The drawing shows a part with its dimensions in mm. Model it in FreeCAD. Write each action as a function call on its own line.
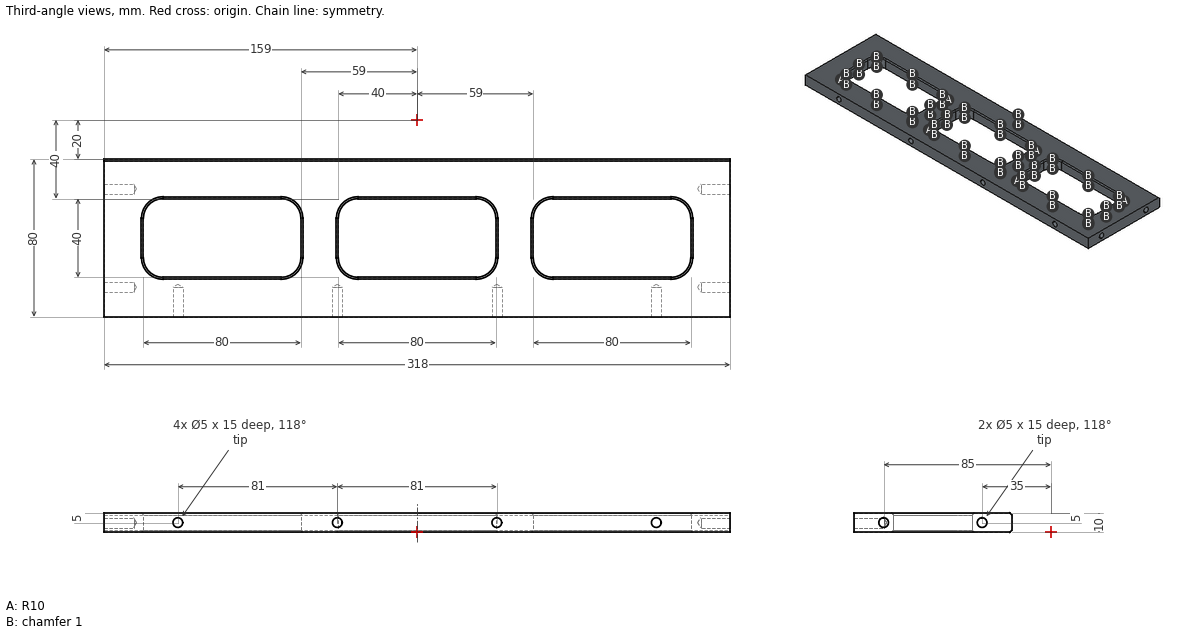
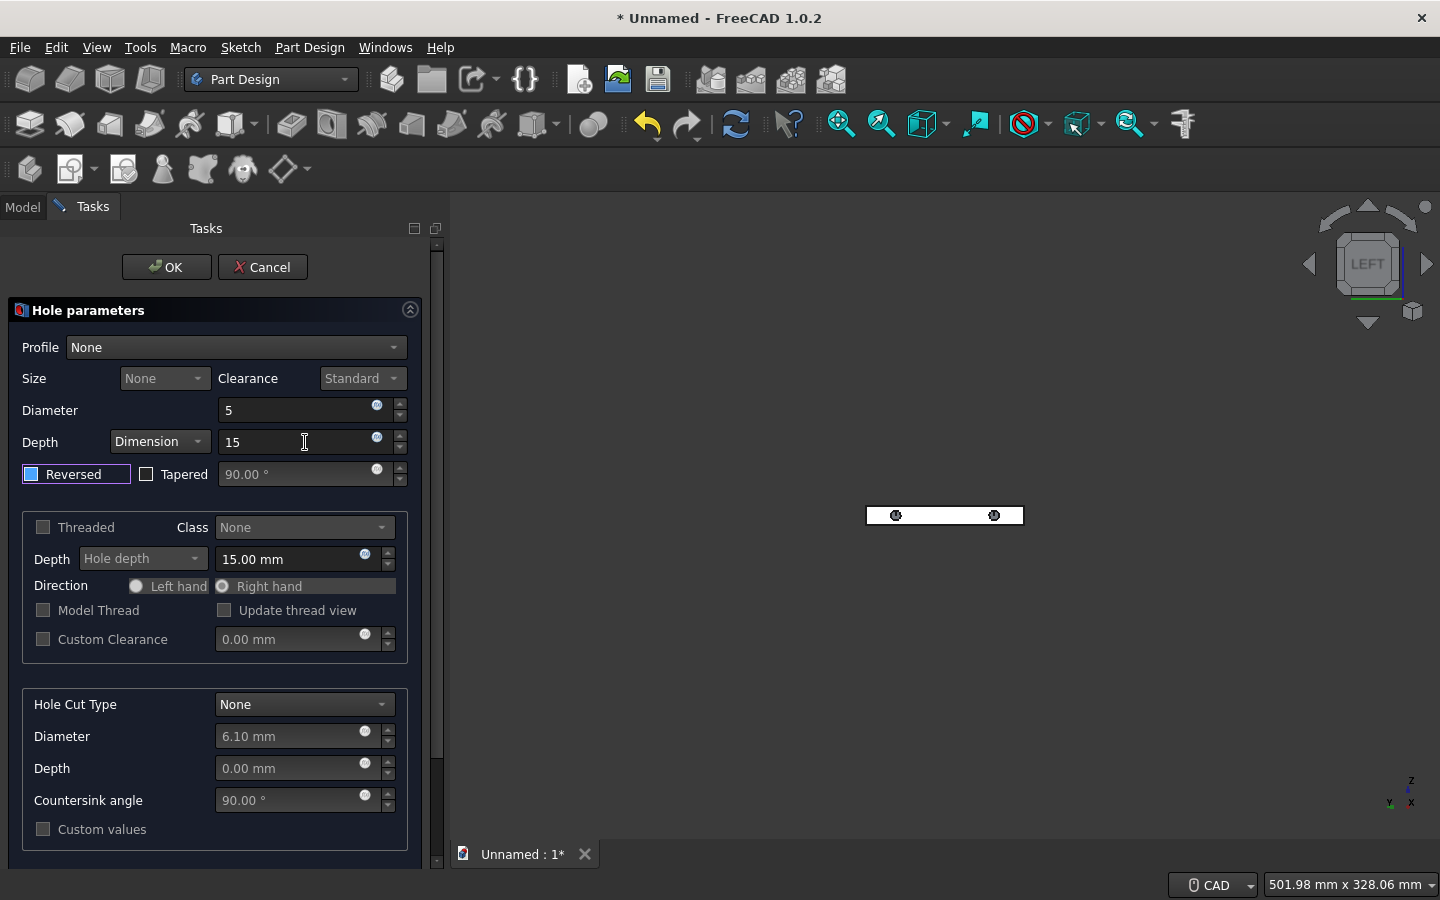
click(167, 267)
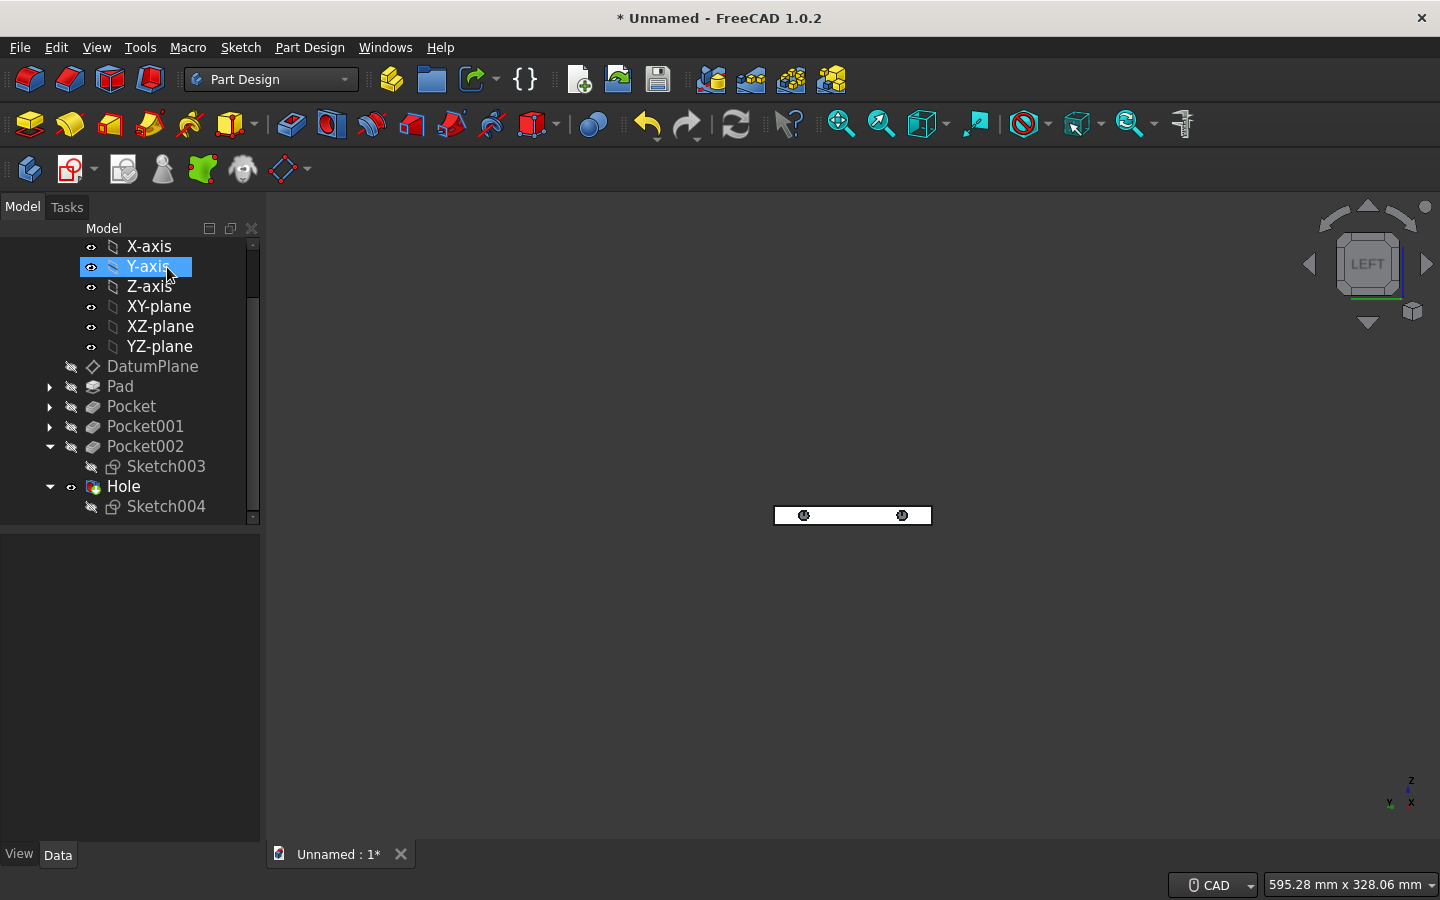
click(842, 124)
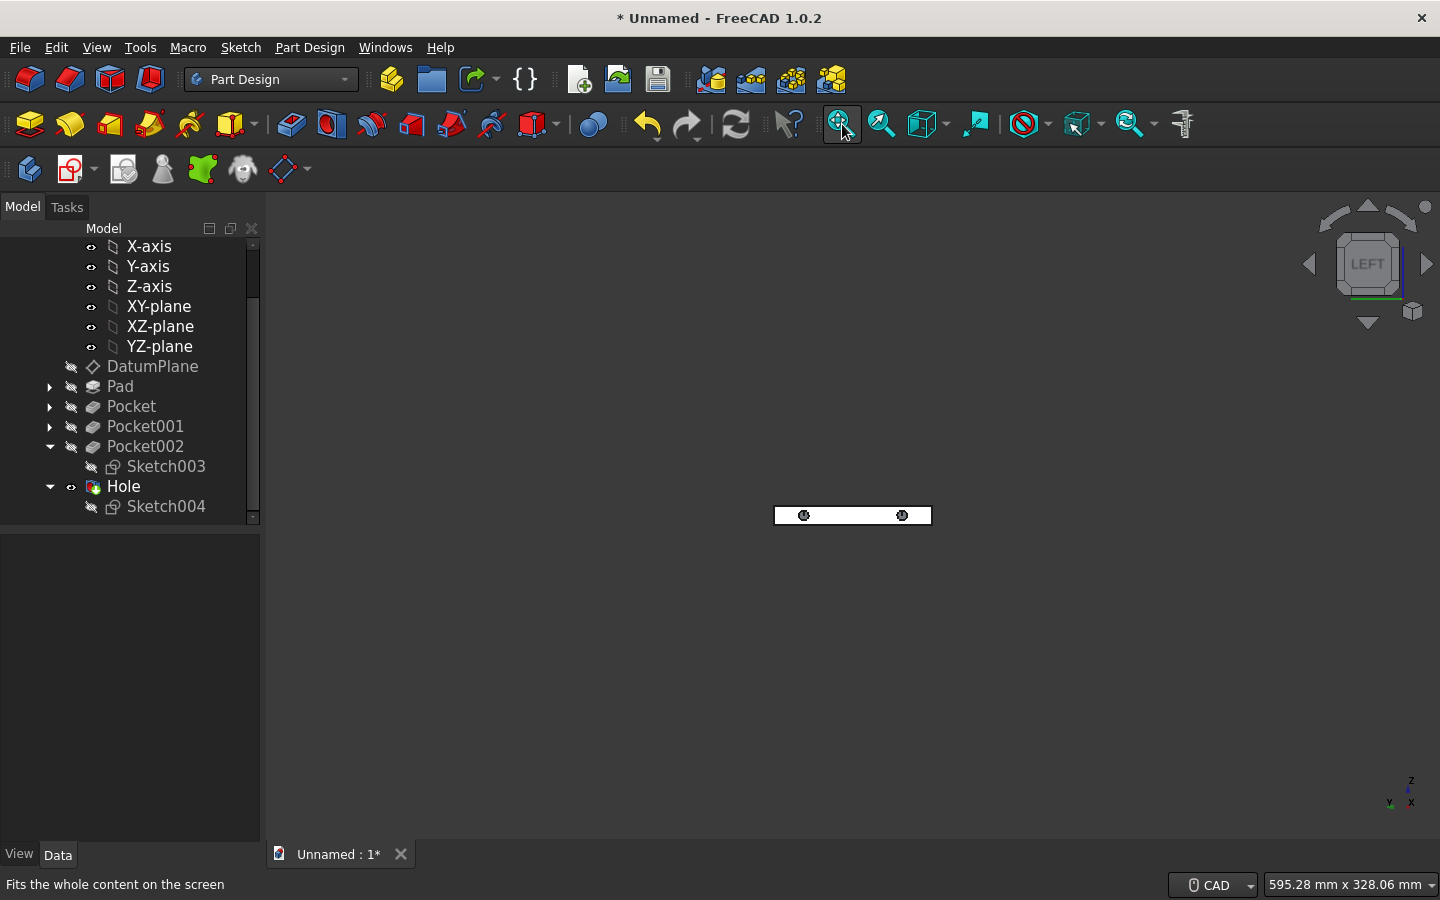
key(0)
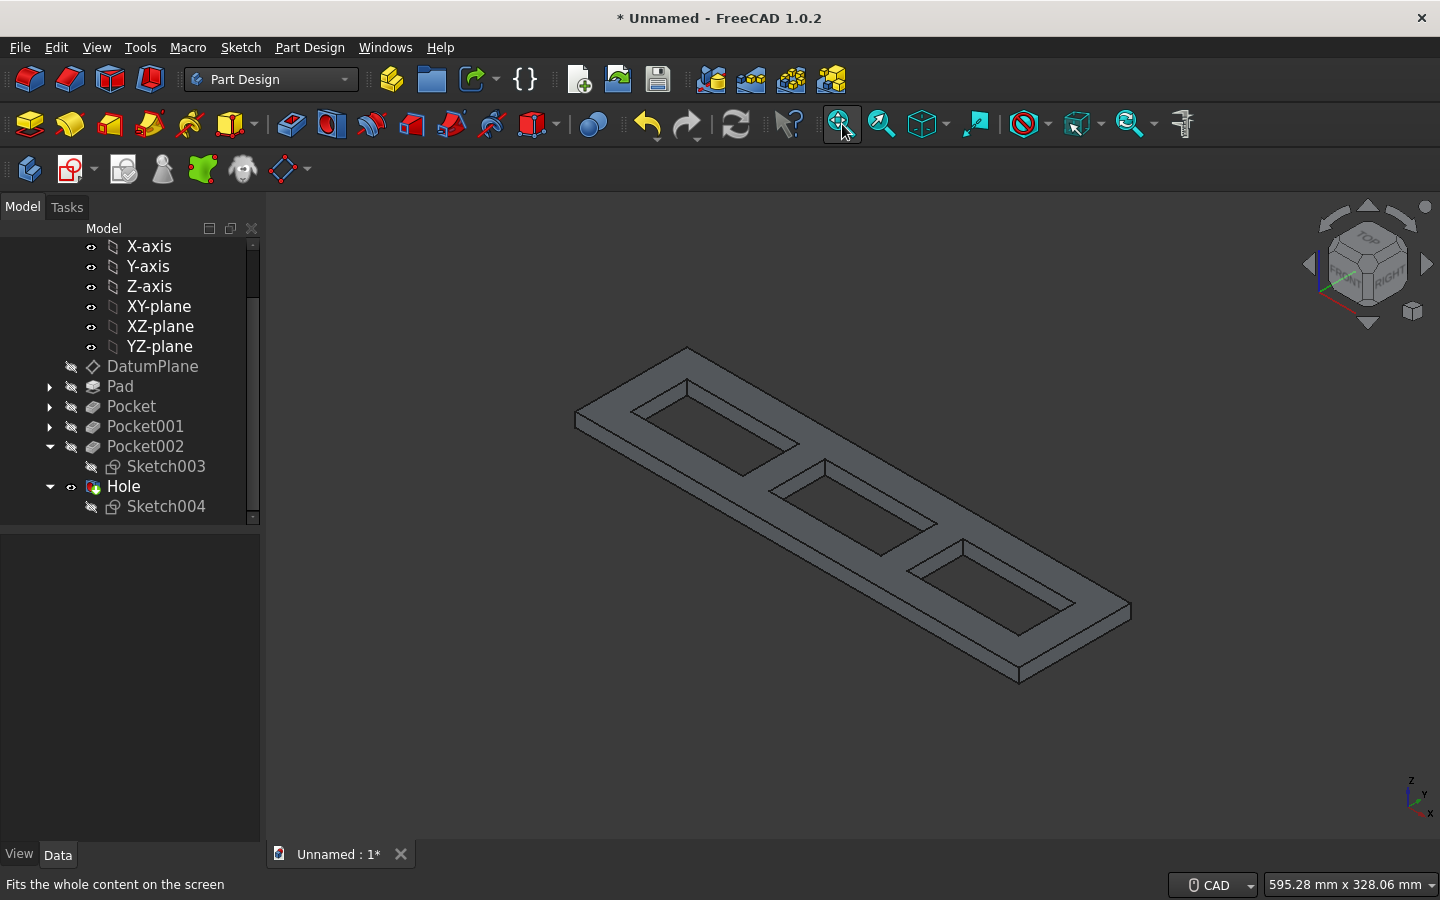
key(3)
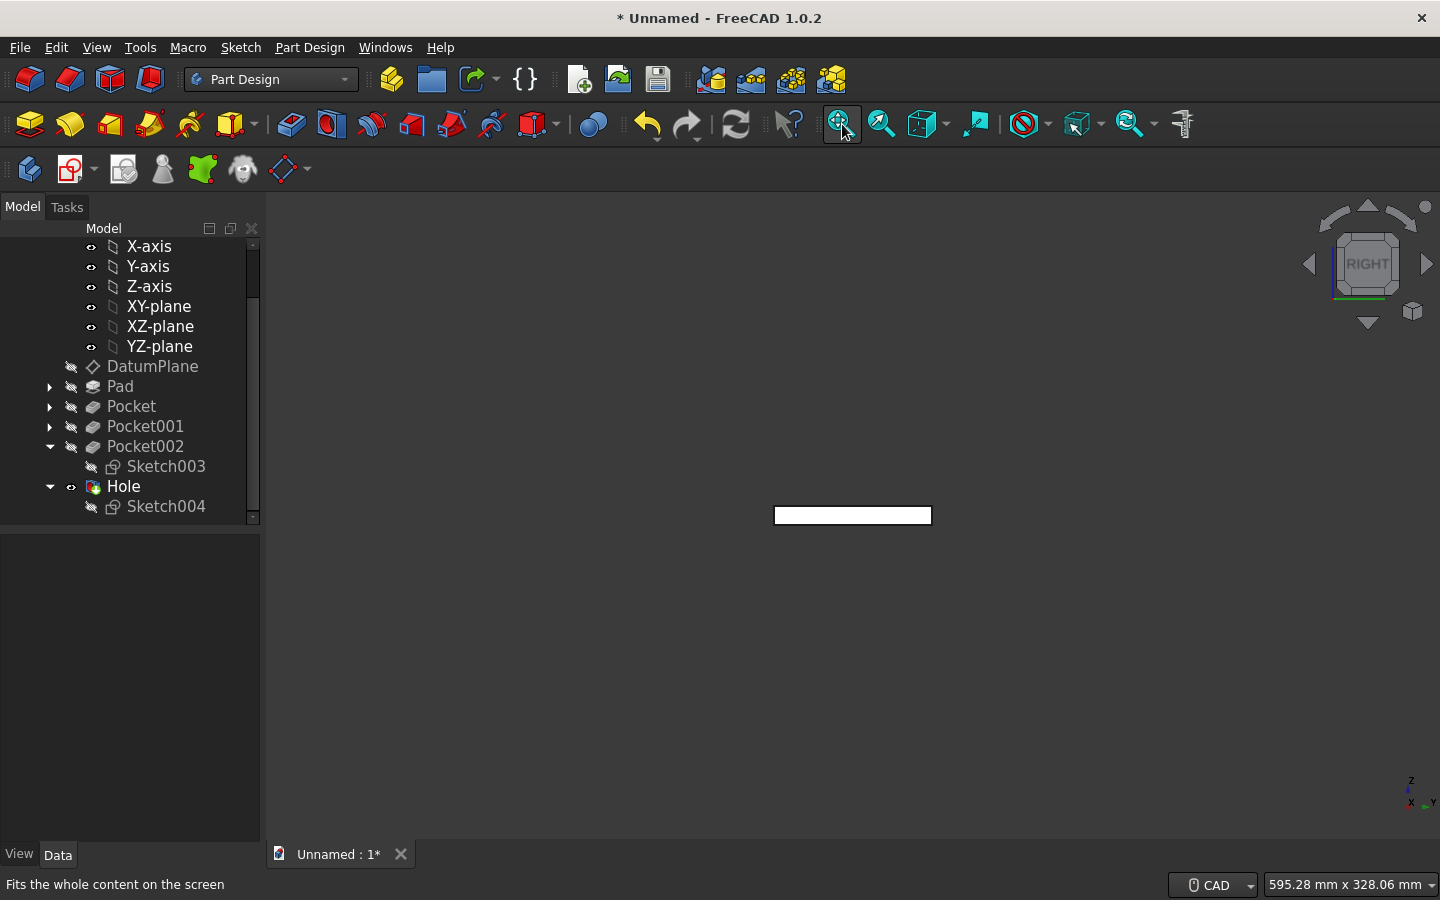
click(842, 124)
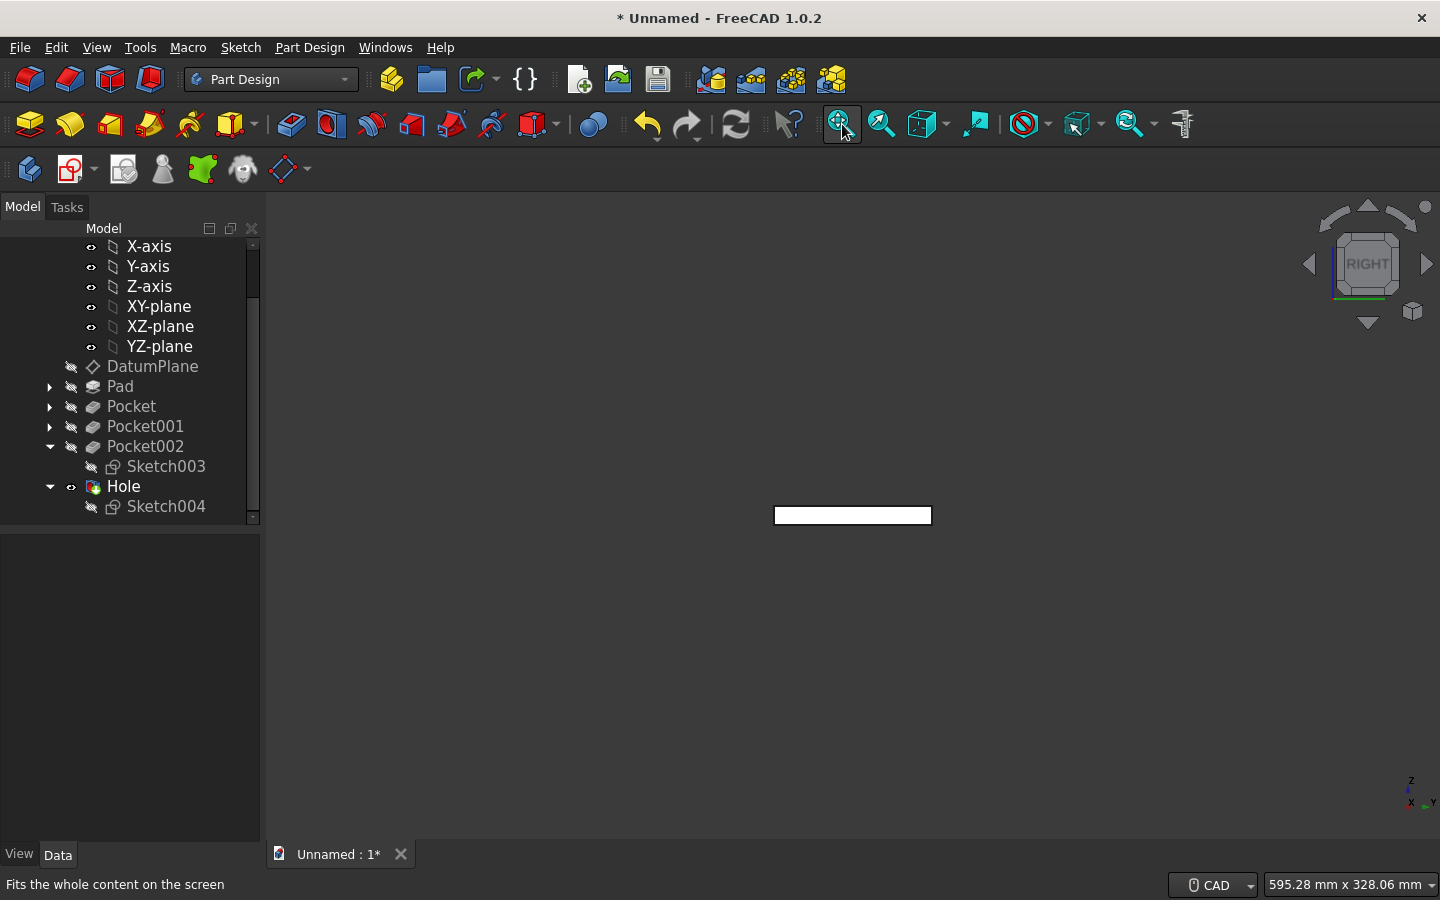
click(921, 514)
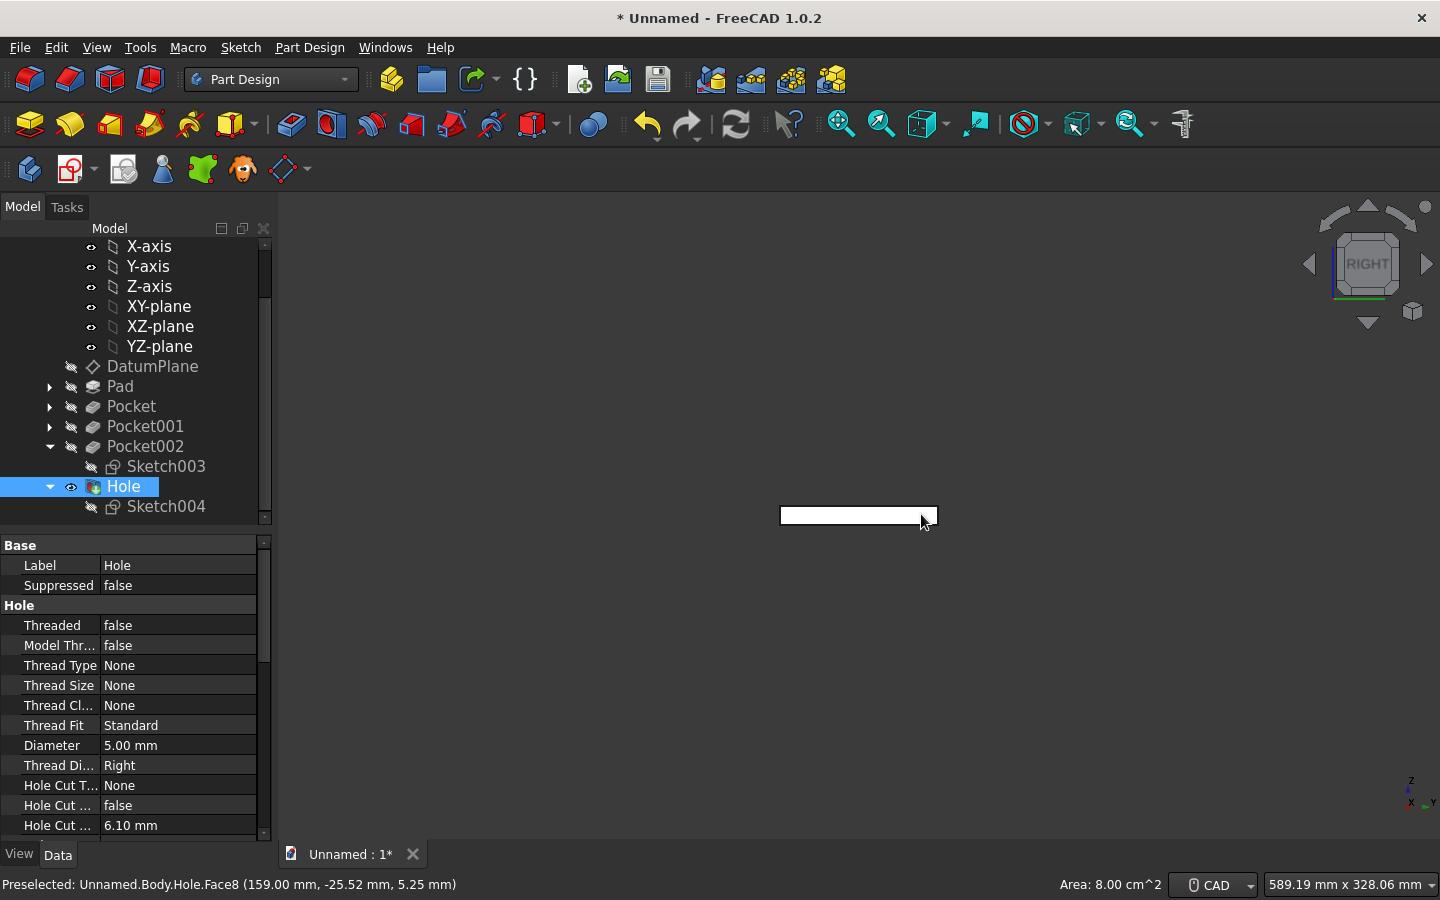
click(70, 170)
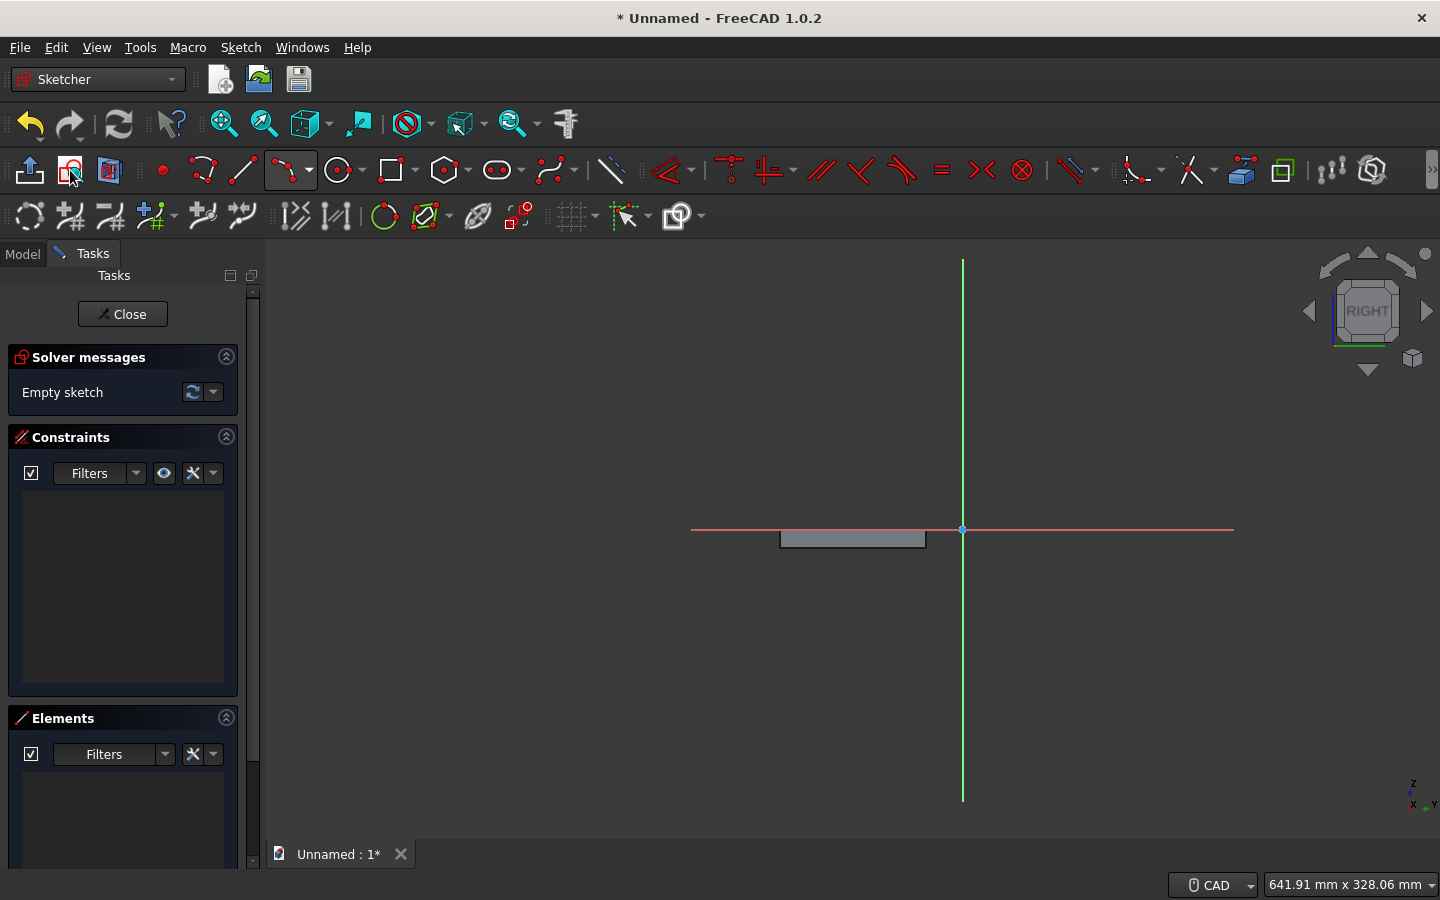
scroll(915, 536, up, 7)